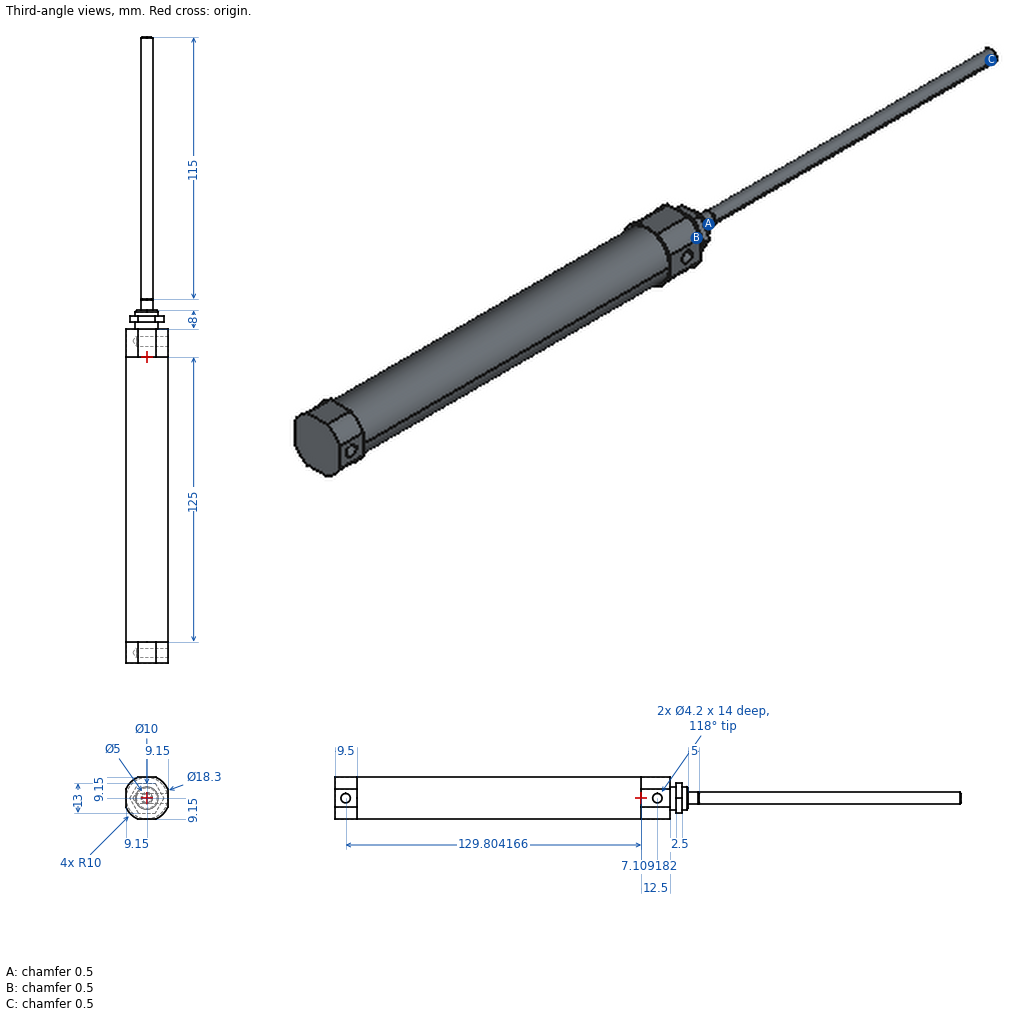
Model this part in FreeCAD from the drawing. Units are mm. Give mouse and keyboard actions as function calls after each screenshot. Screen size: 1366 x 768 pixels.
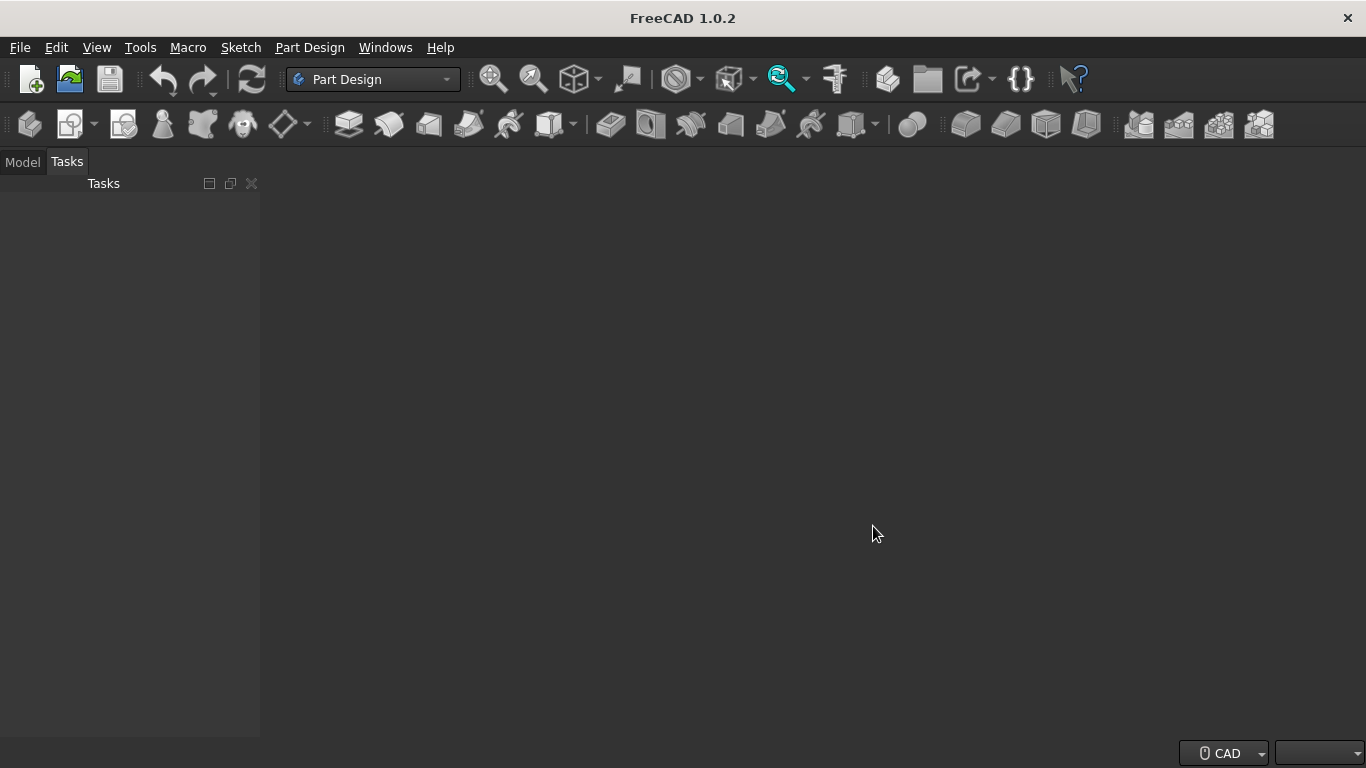
key(ctrl+n)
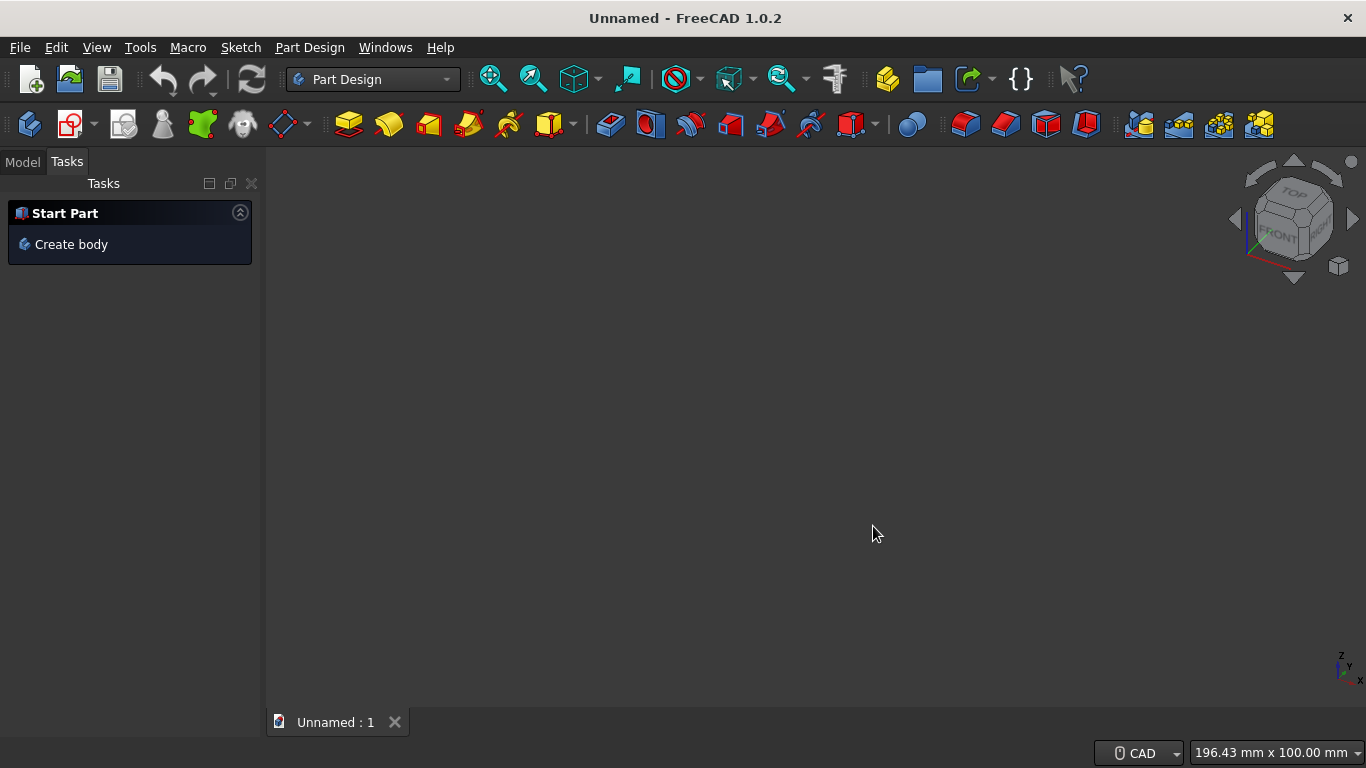
click(70, 124)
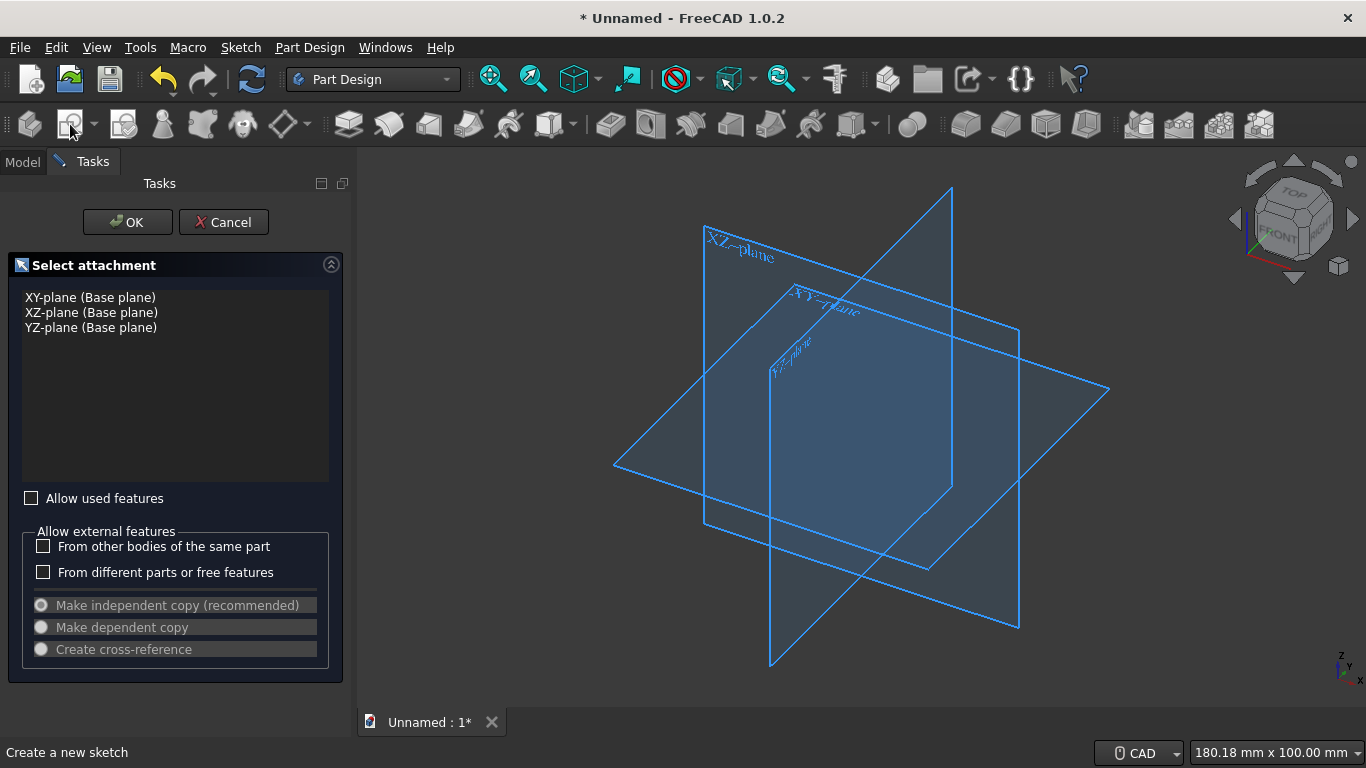
click(82, 312)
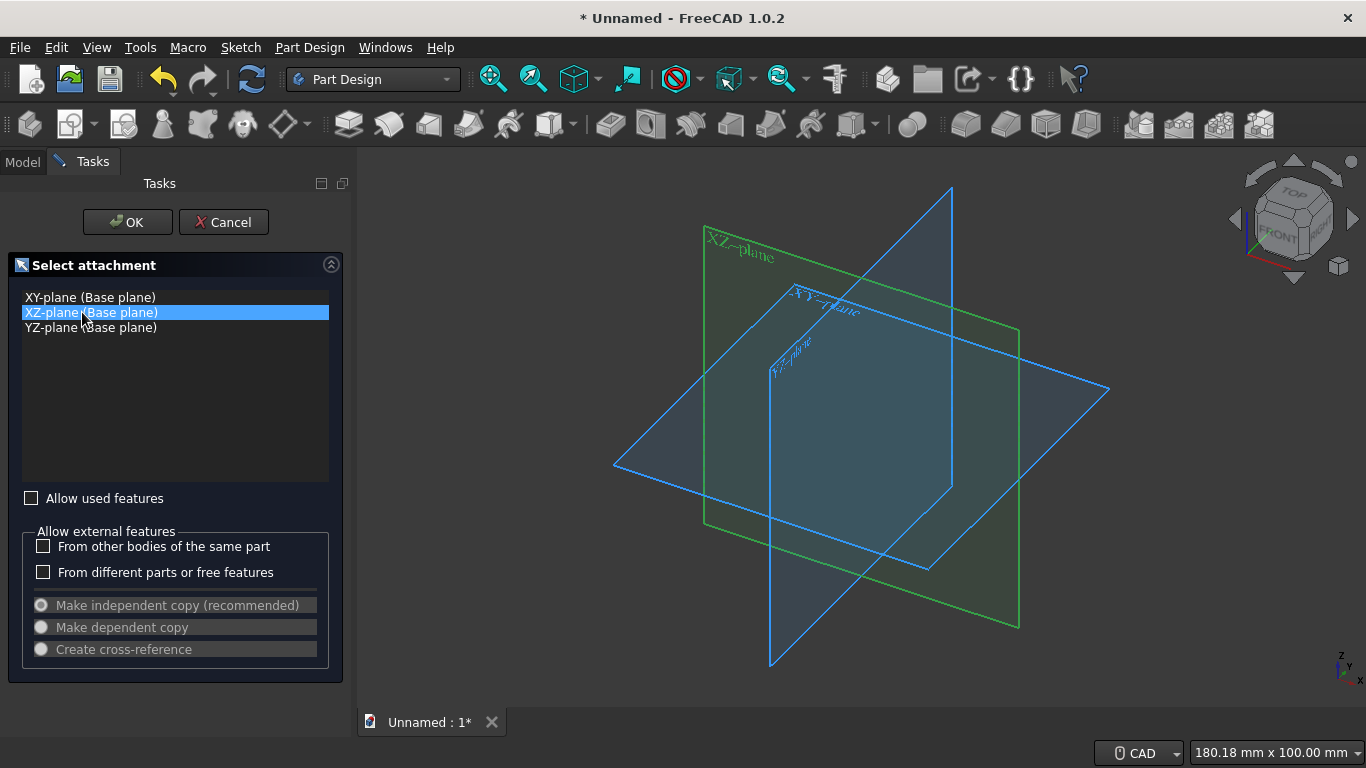
click(128, 222)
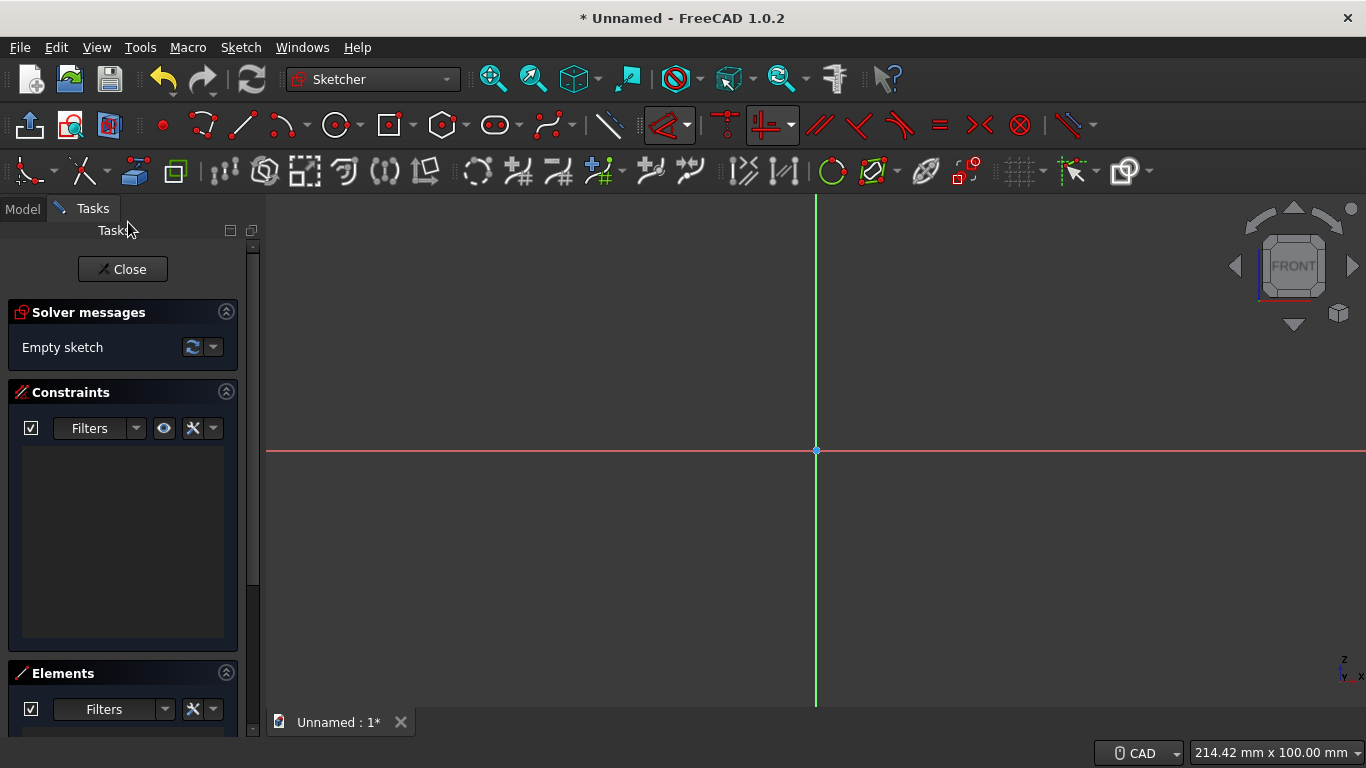
scroll(846, 450, up, 6)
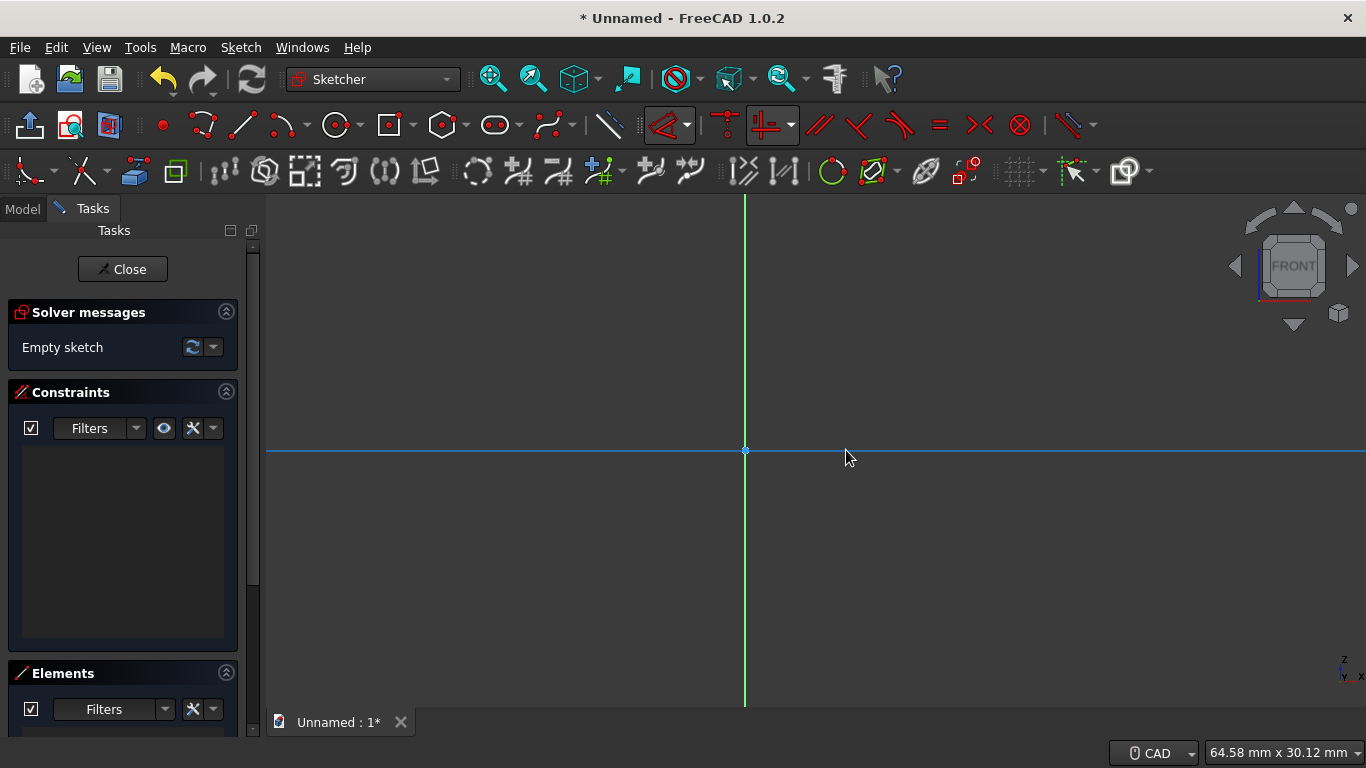
click(244, 126)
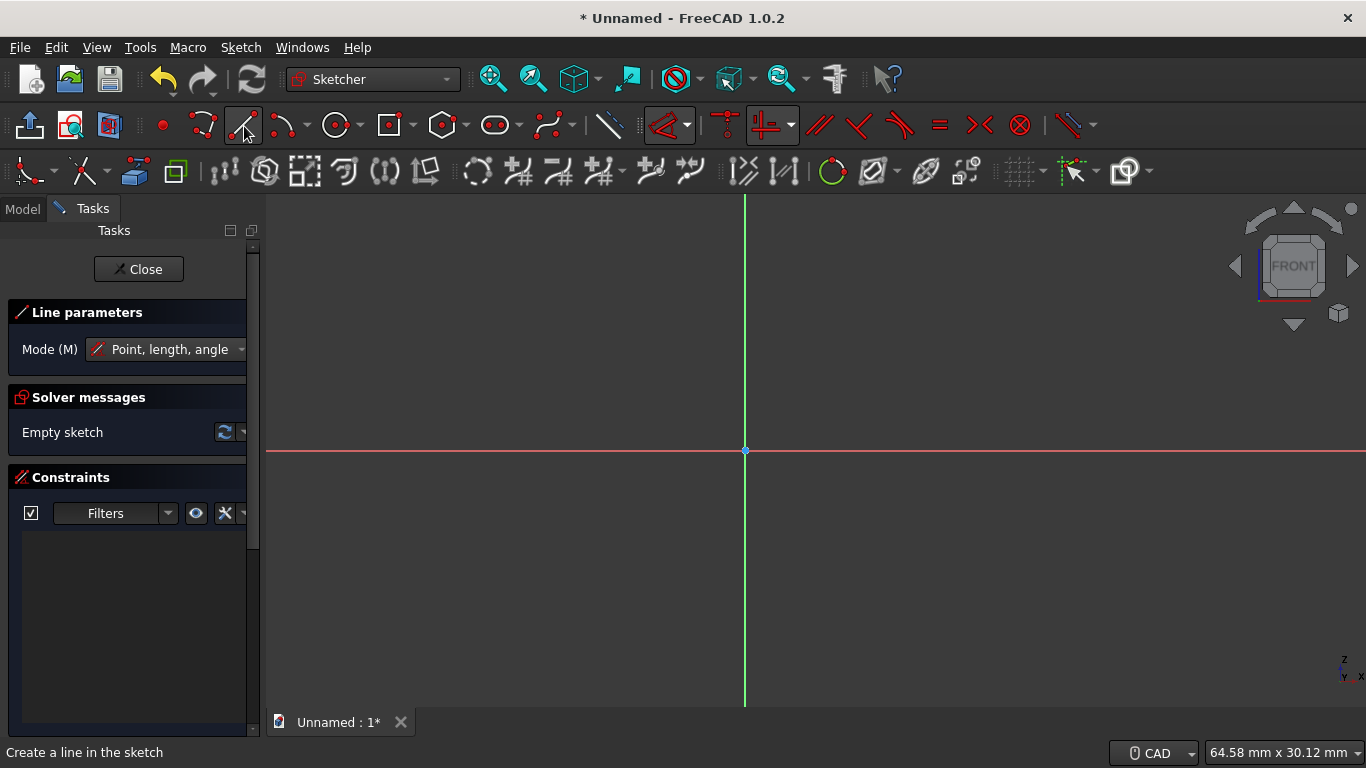
click(814, 606)
click(676, 606)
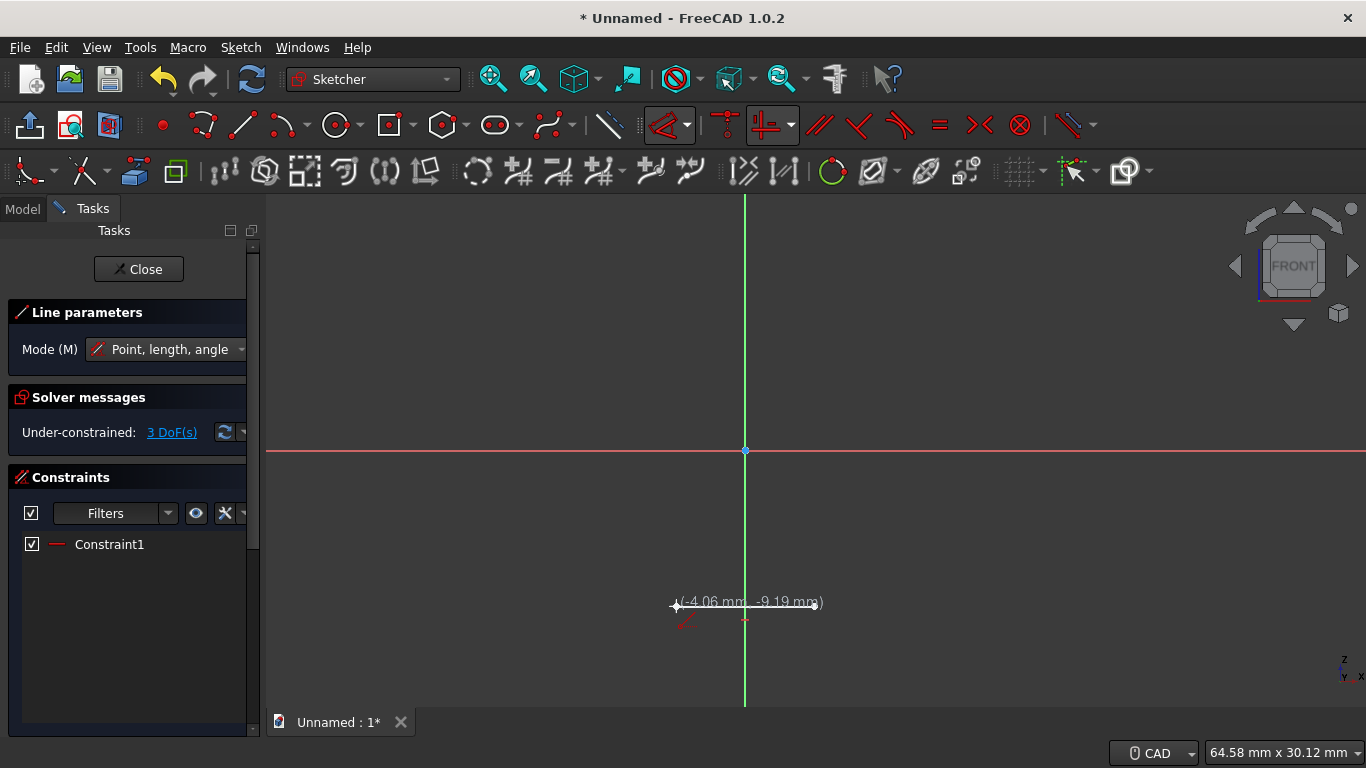
click(589, 519)
click(589, 382)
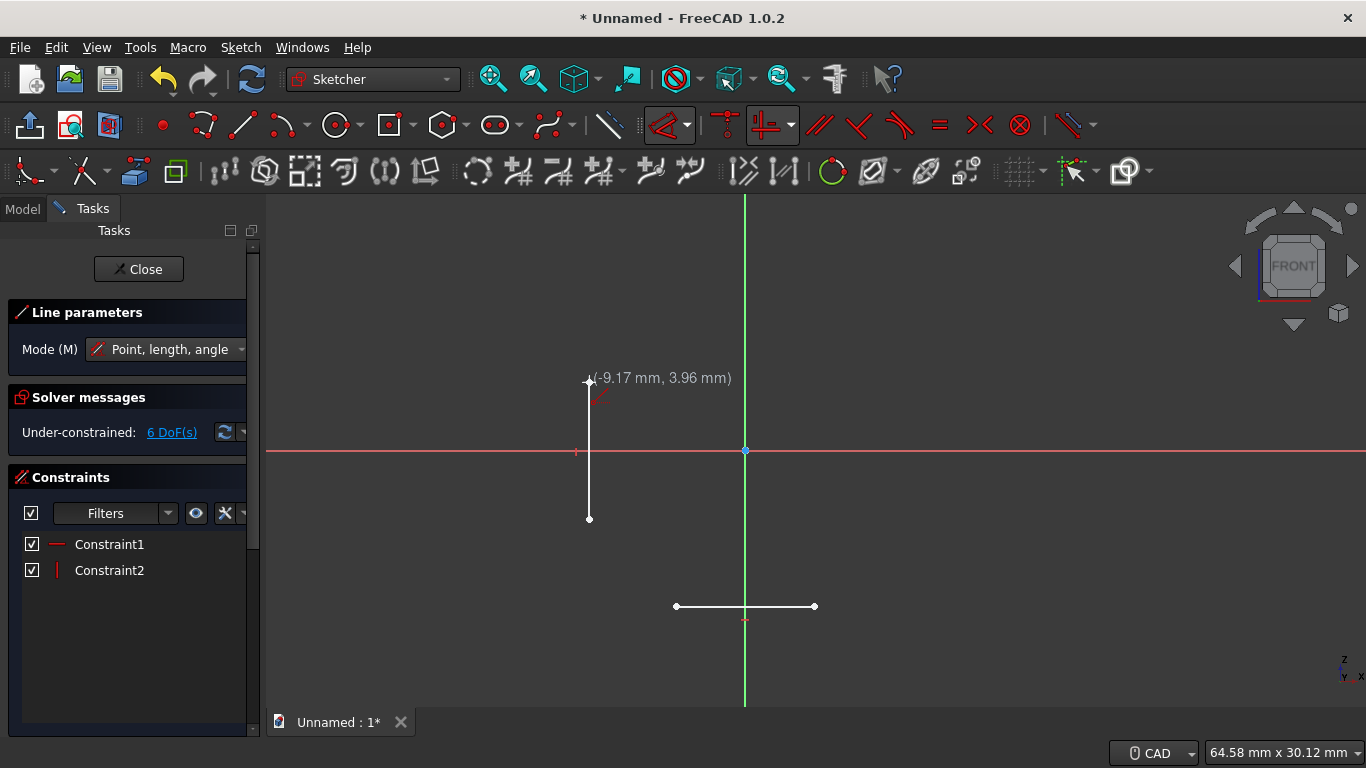
click(676, 295)
click(814, 295)